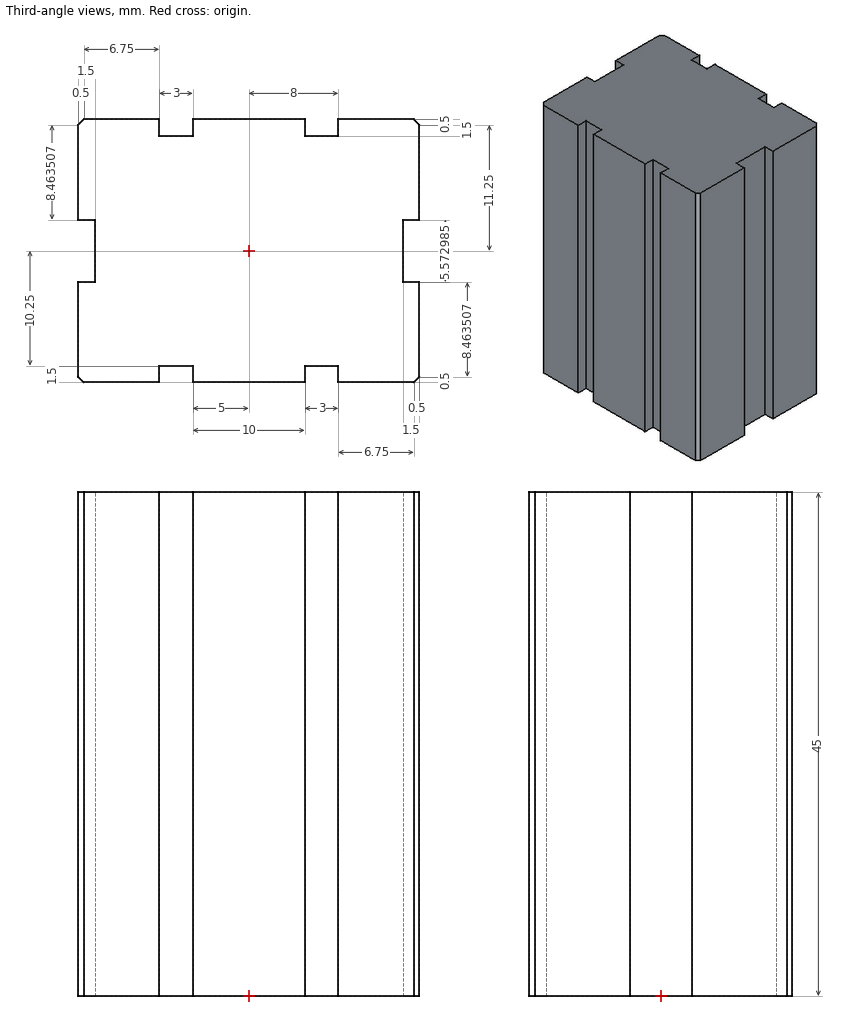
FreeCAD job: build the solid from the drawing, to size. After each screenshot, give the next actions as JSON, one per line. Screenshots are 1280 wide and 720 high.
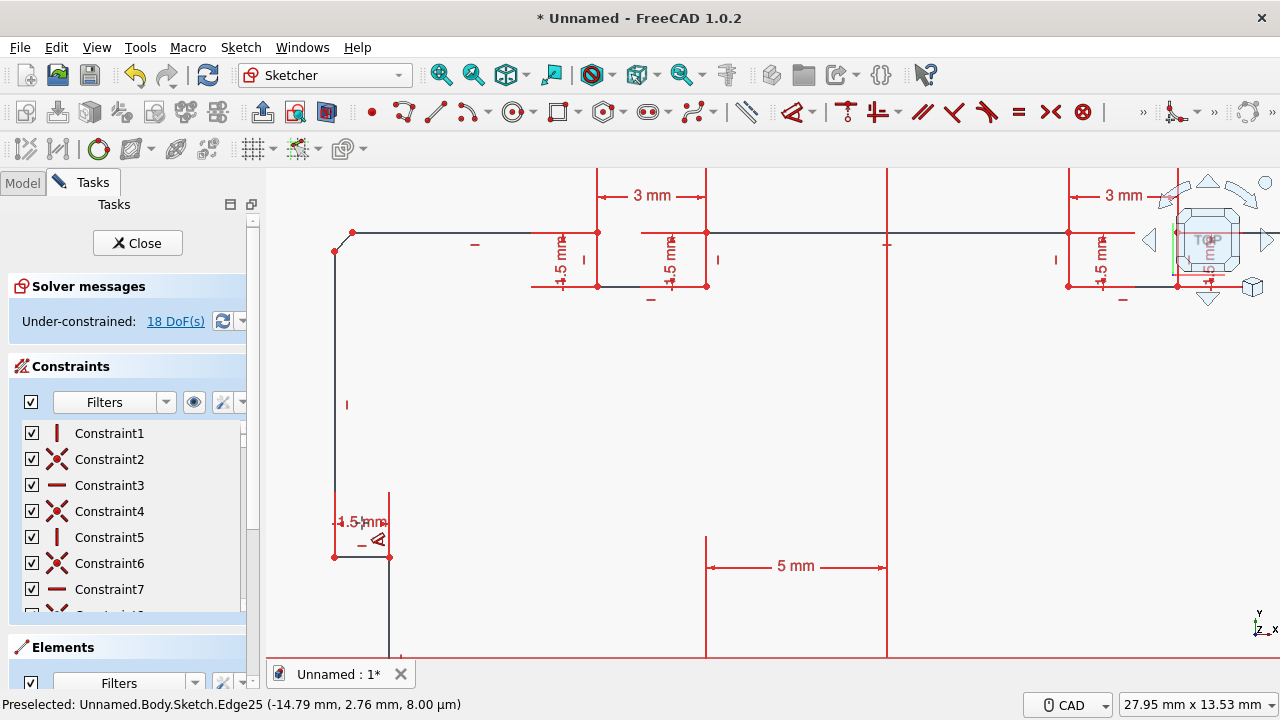
{"action": "scroll", "coordinate": [598, 271], "scroll_direction": "down", "scroll_amount": 5}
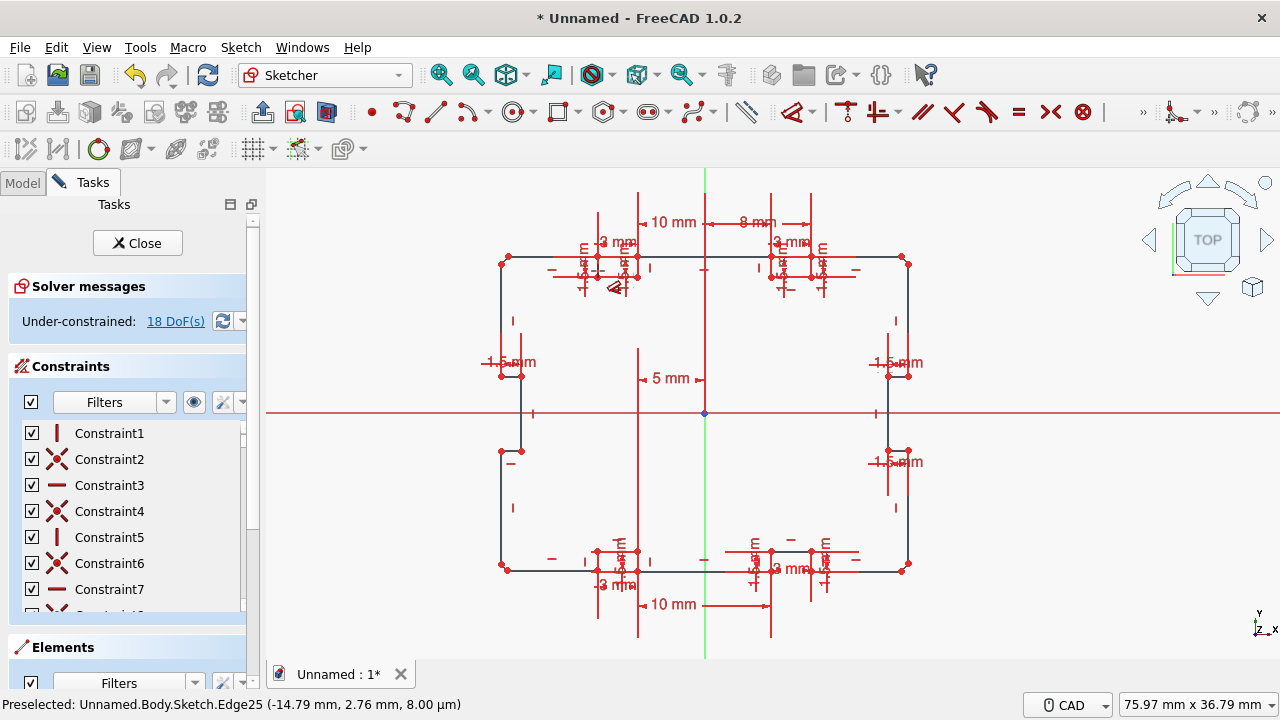
{"action": "scroll", "coordinate": [515, 451], "scroll_direction": "up", "scroll_amount": 5}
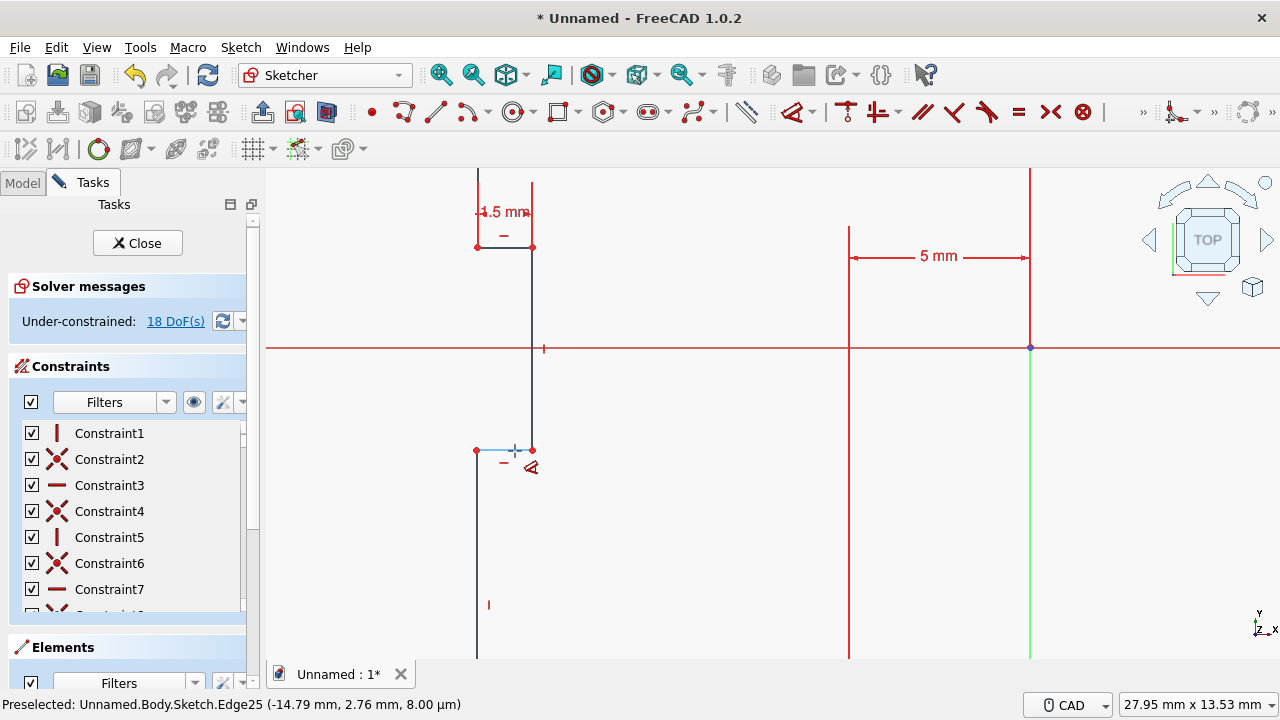
{"action": "left_click", "coordinate": [515, 450]}
{"action": "left_click", "coordinate": [504, 484]}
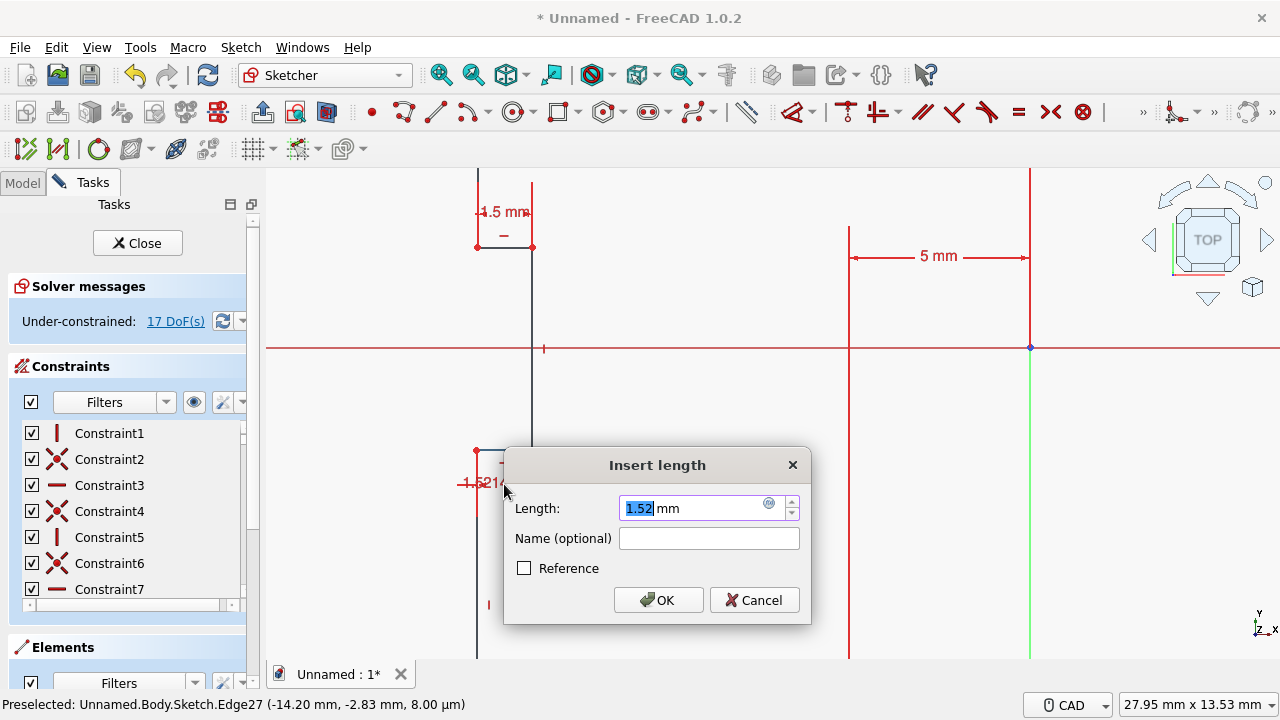
{"action": "type", "text": "1.5"}
{"action": "key", "text": "Return"}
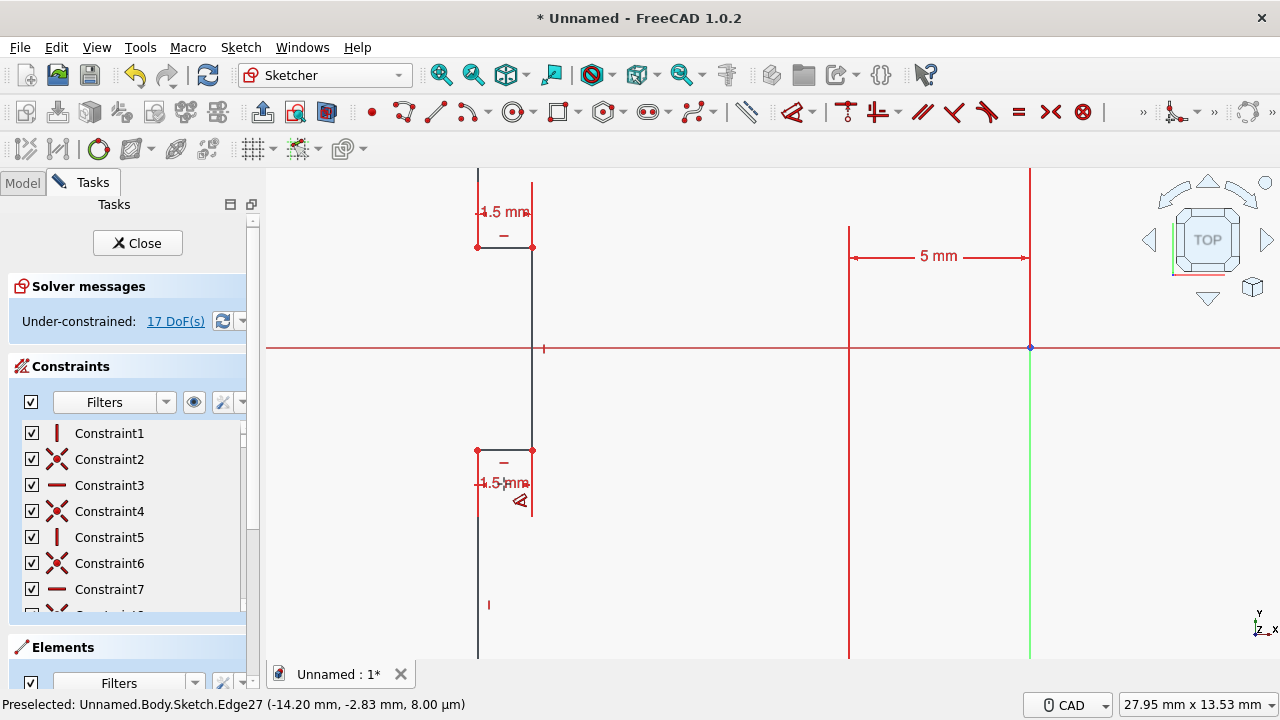
{"action": "scroll", "coordinate": [515, 452], "scroll_direction": "down", "scroll_amount": 5}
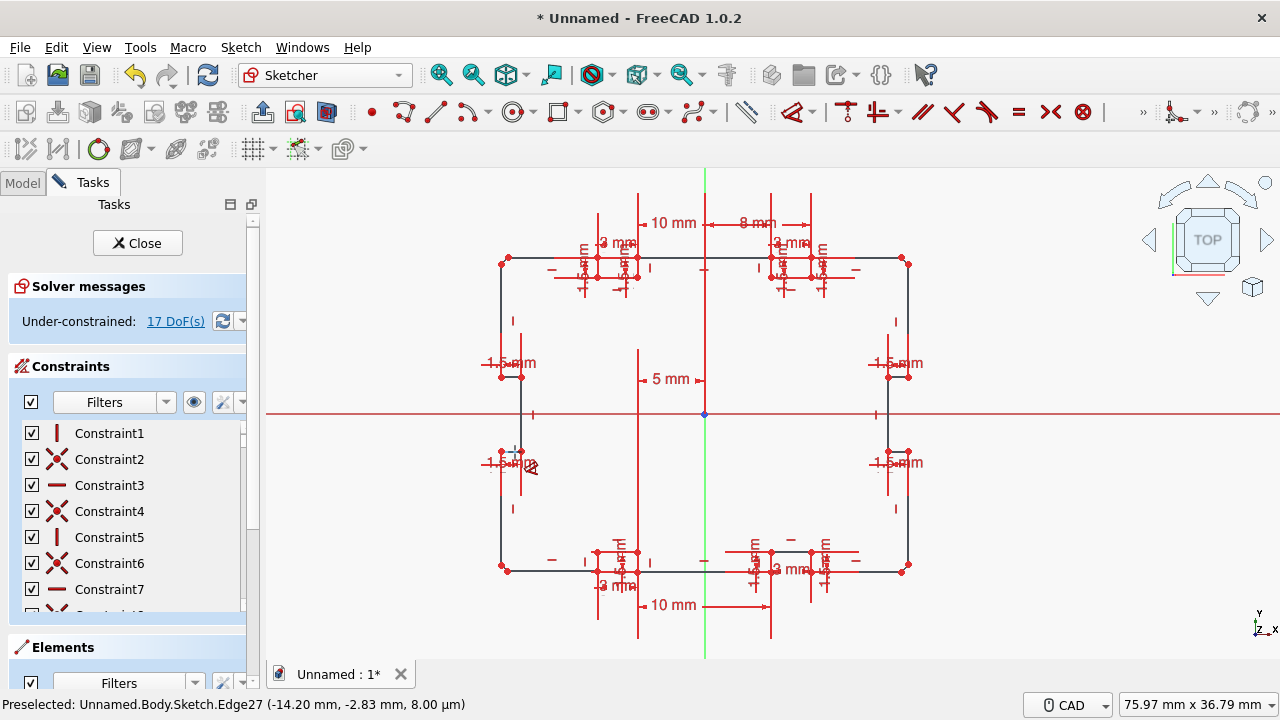
{"action": "scroll", "coordinate": [598, 566], "scroll_direction": "up", "scroll_amount": 5}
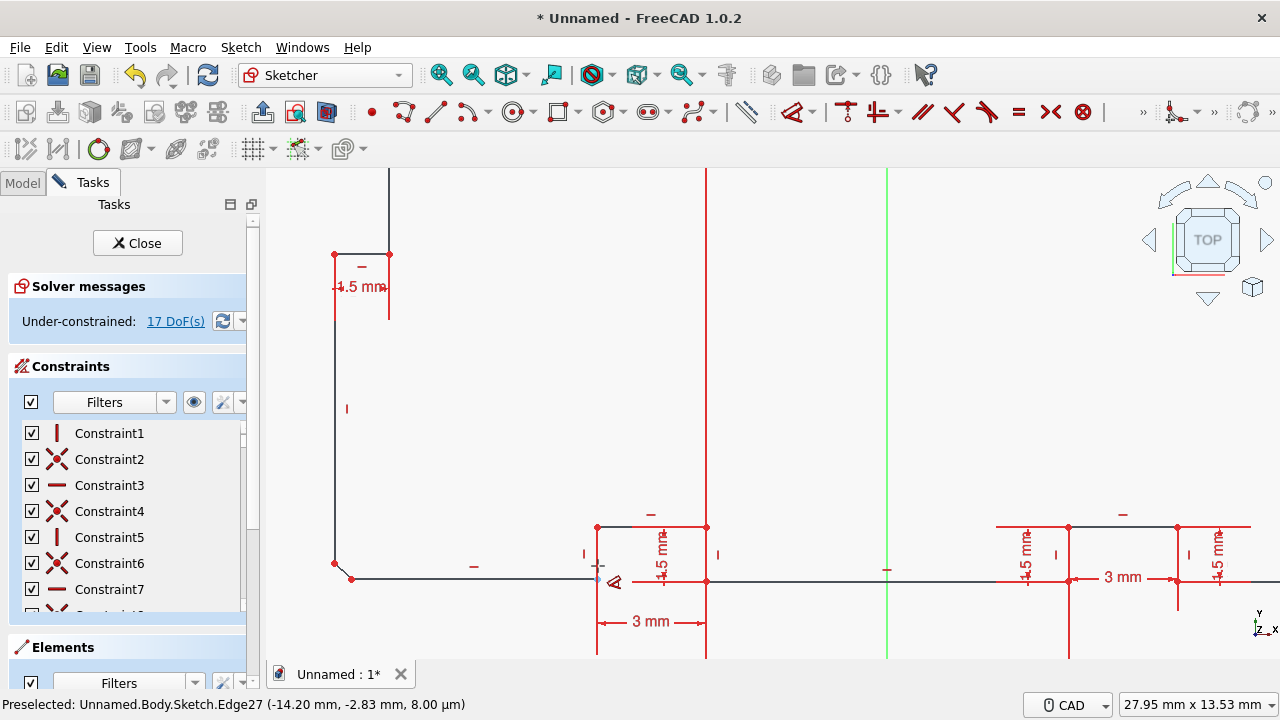
{"action": "left_click", "coordinate": [597, 564]}
{"action": "left_click", "coordinate": [563, 553]}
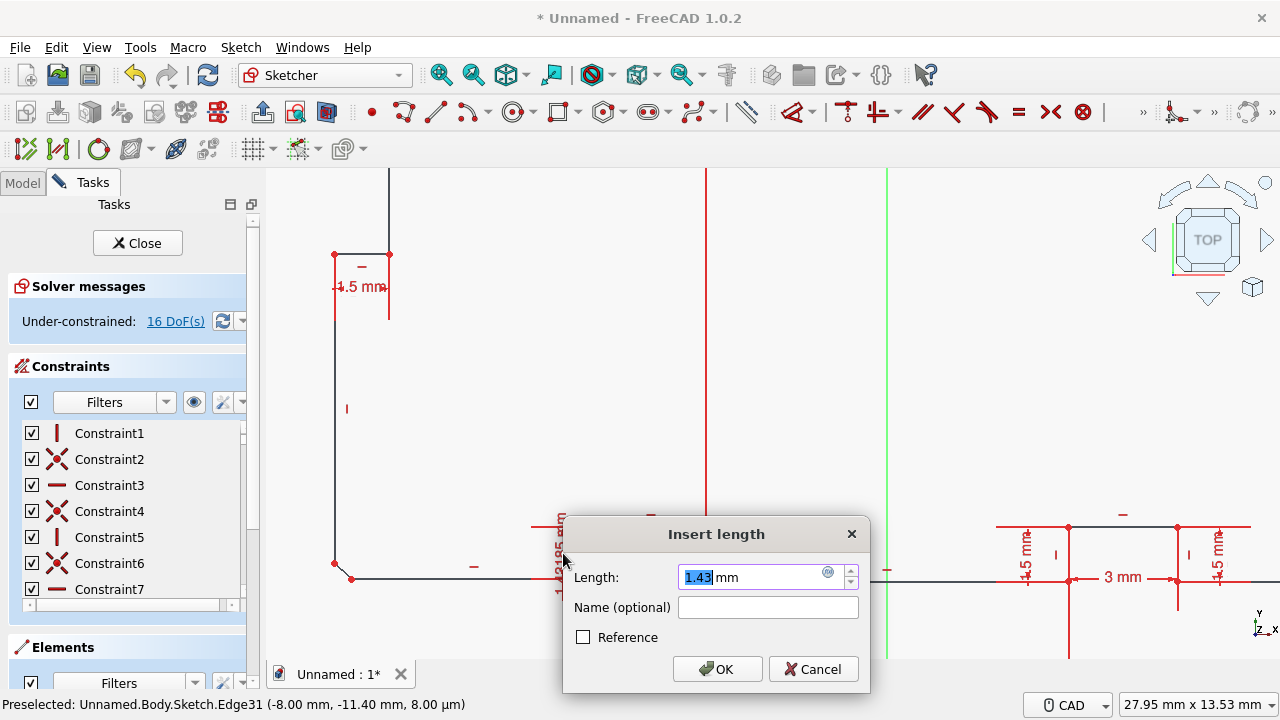
{"action": "type", "text": "1.5"}
{"action": "key", "text": "Return"}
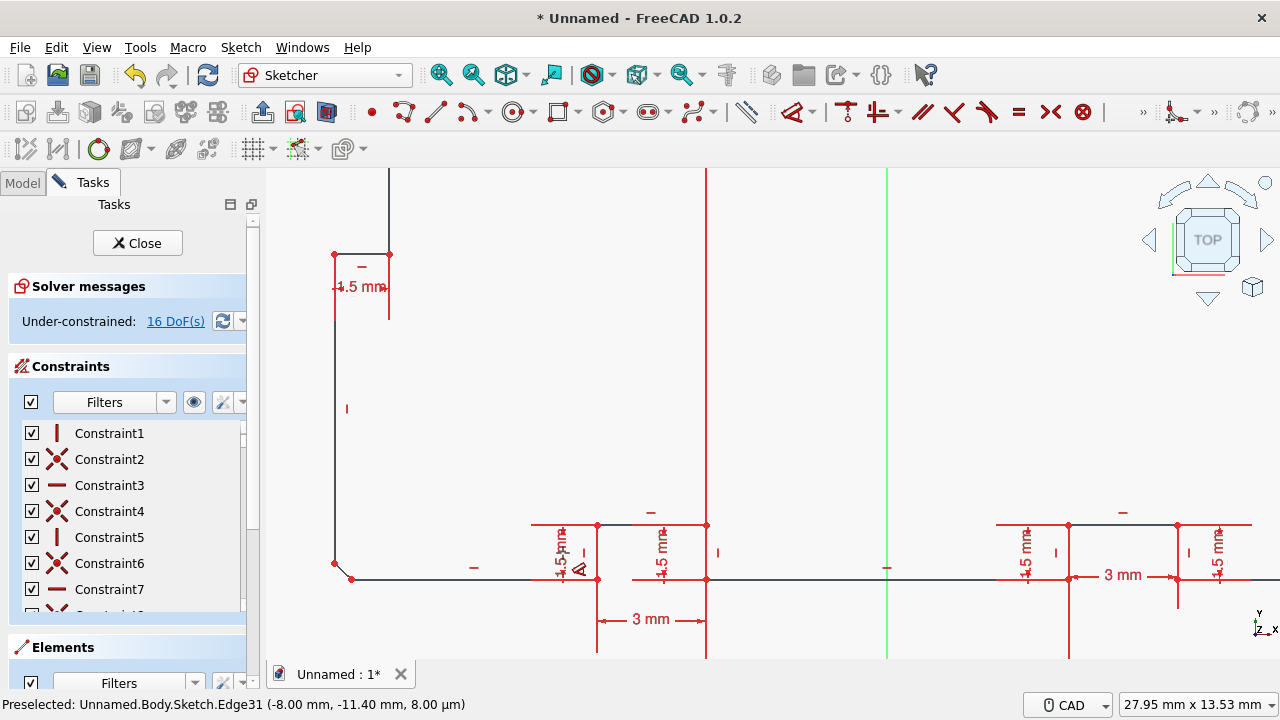
{"action": "scroll", "coordinate": [598, 566], "scroll_direction": "down", "scroll_amount": 5}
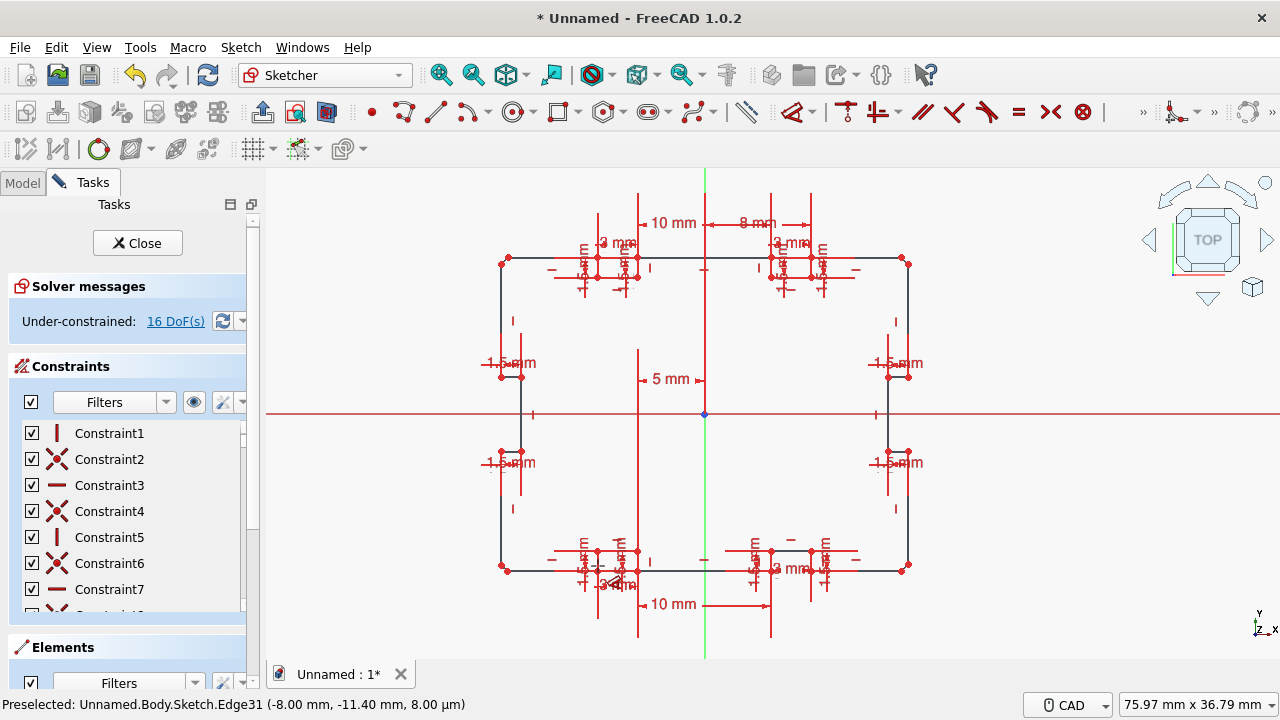
{"action": "left_click", "coordinate": [838, 571]}
{"action": "left_click", "coordinate": [856, 605]}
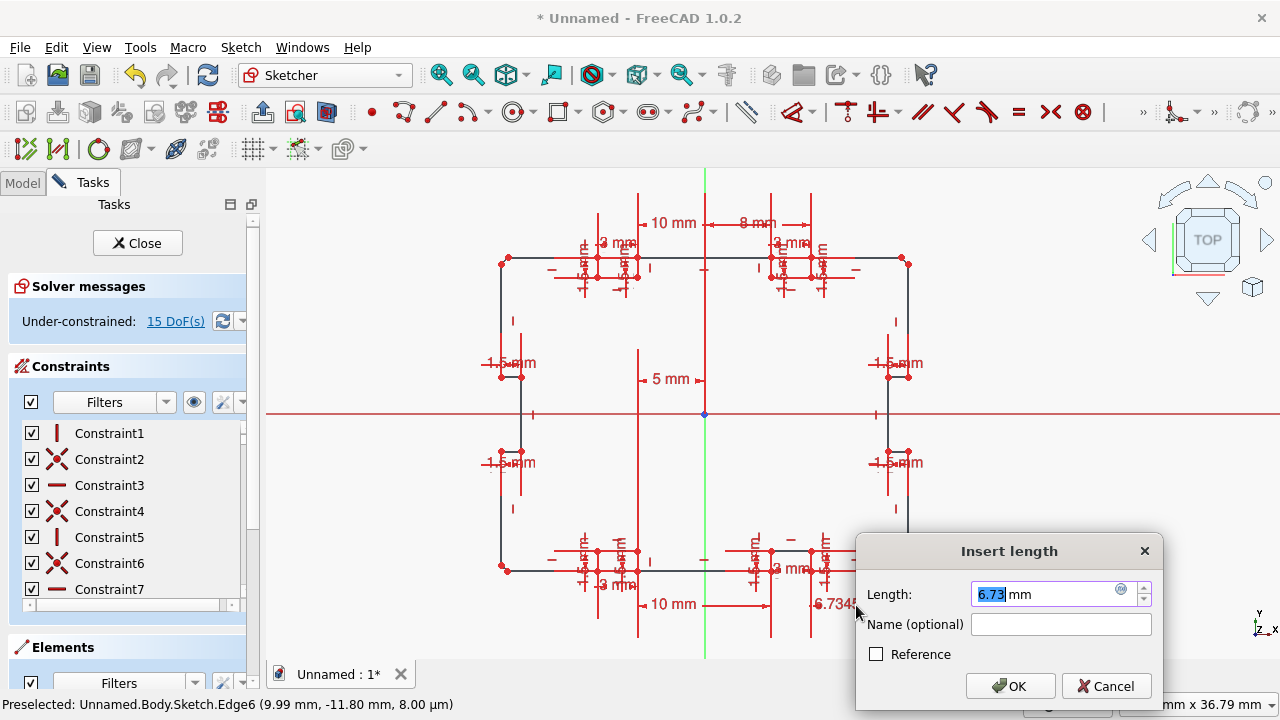
{"action": "type", "text": "6.75"}
{"action": "key", "text": "Return"}